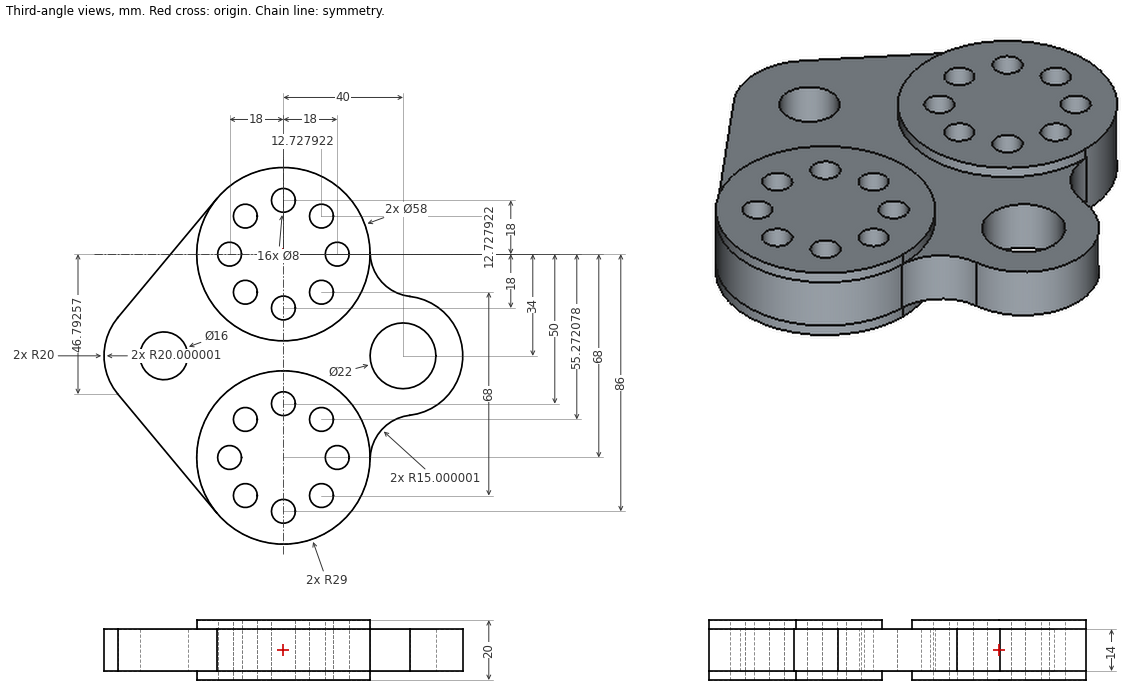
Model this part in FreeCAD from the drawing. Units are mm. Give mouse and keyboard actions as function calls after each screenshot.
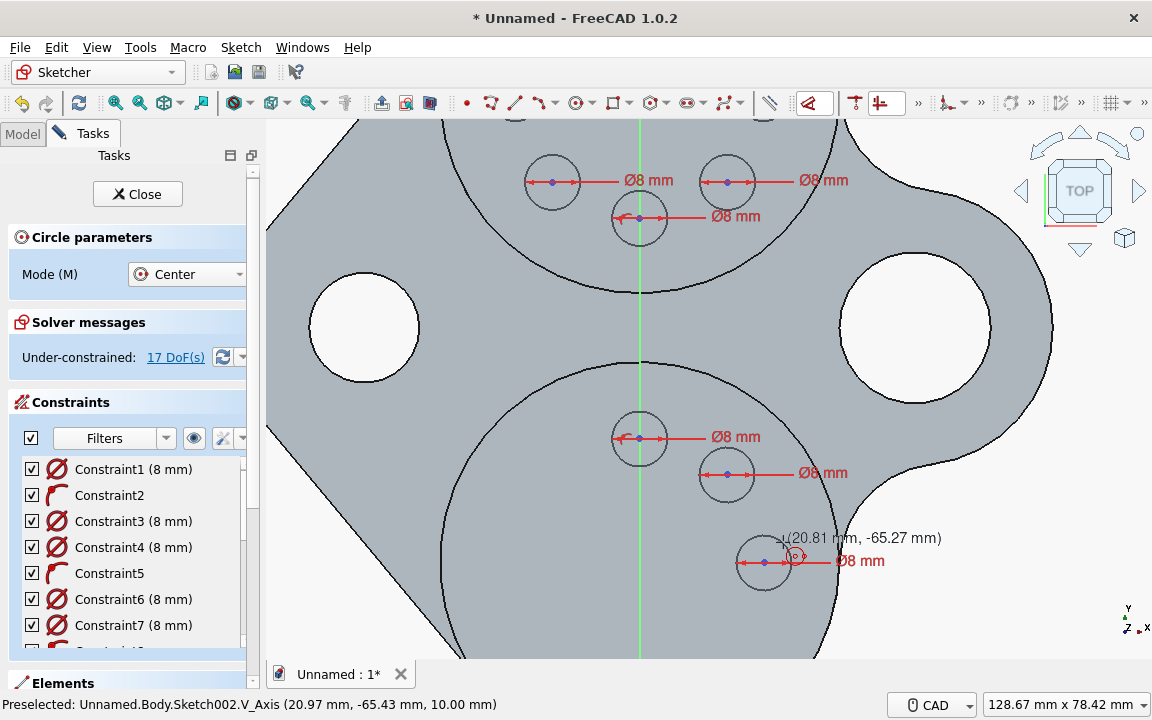
scroll(641, 439, down, 4)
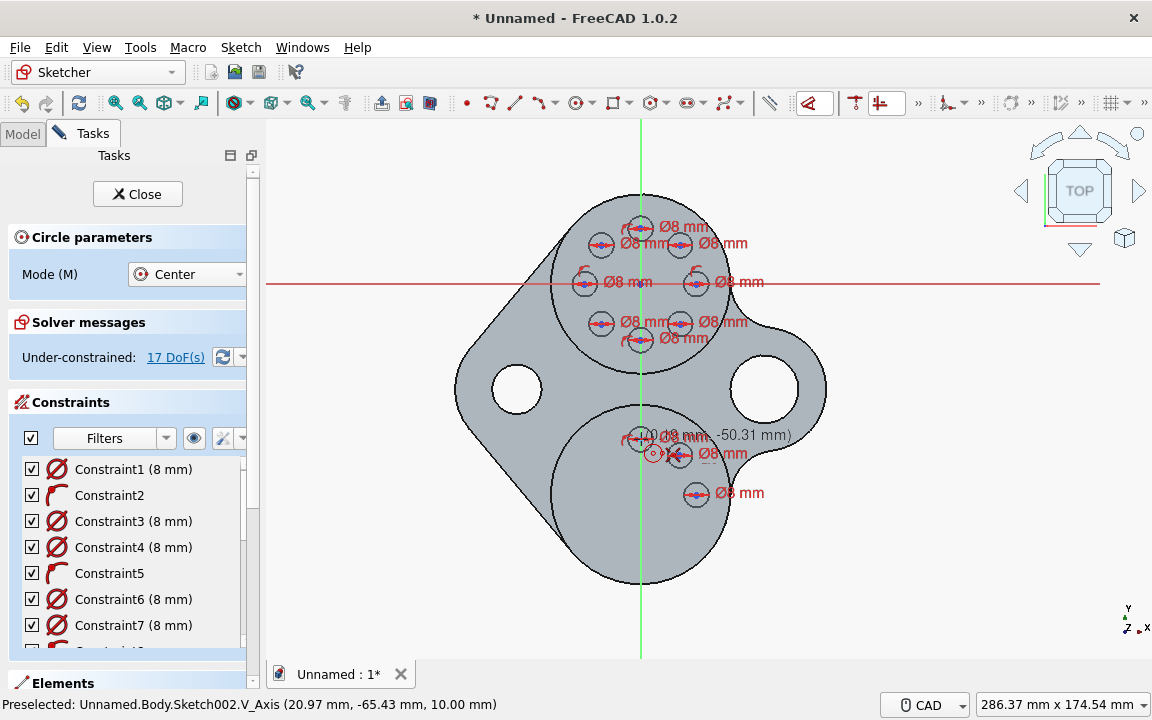
scroll(680, 534, up, 4)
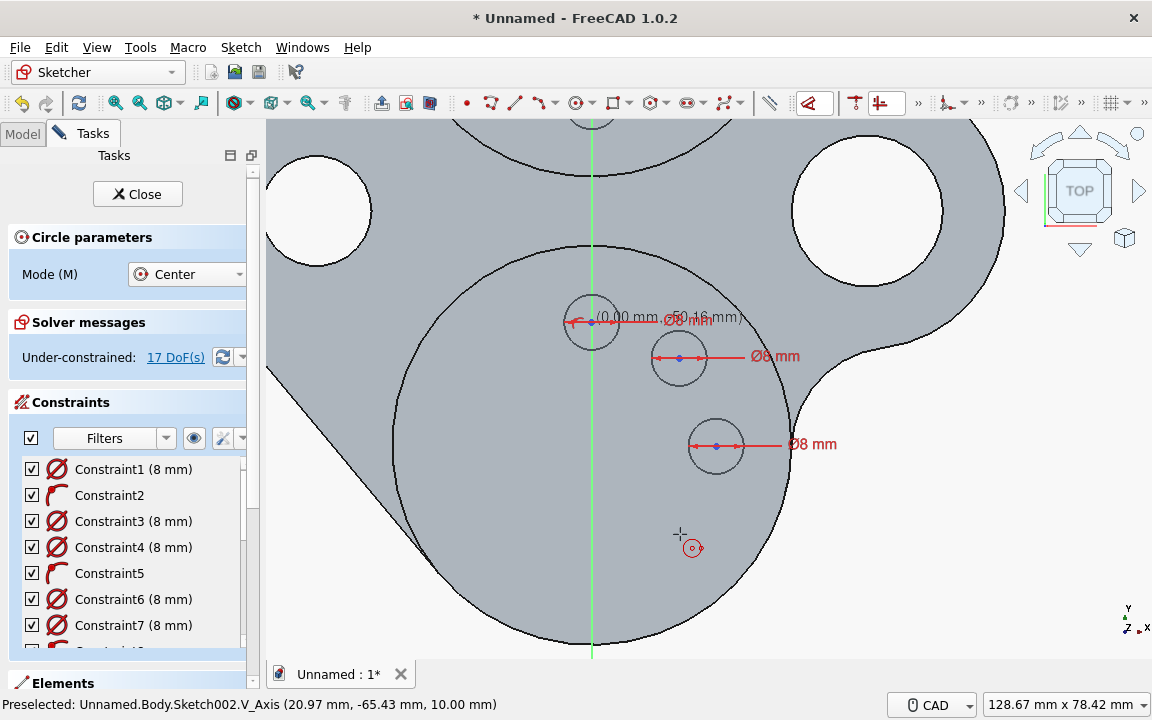
click(679, 533)
move(699, 513)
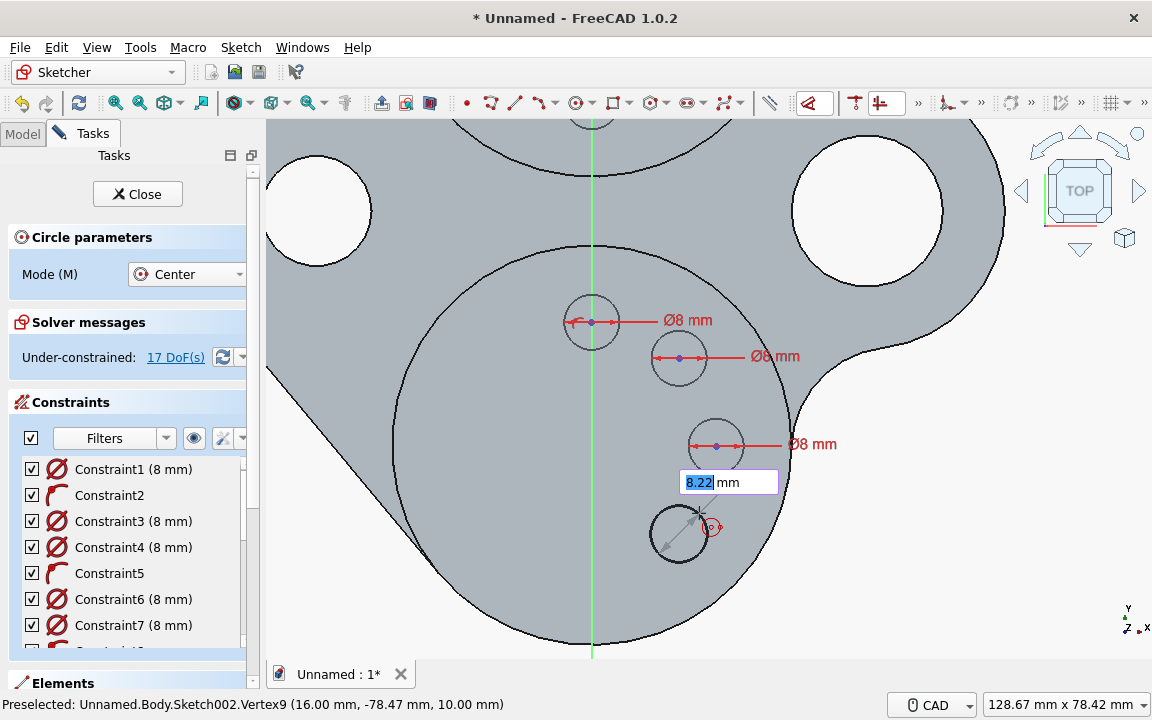
text(8)
key(Return)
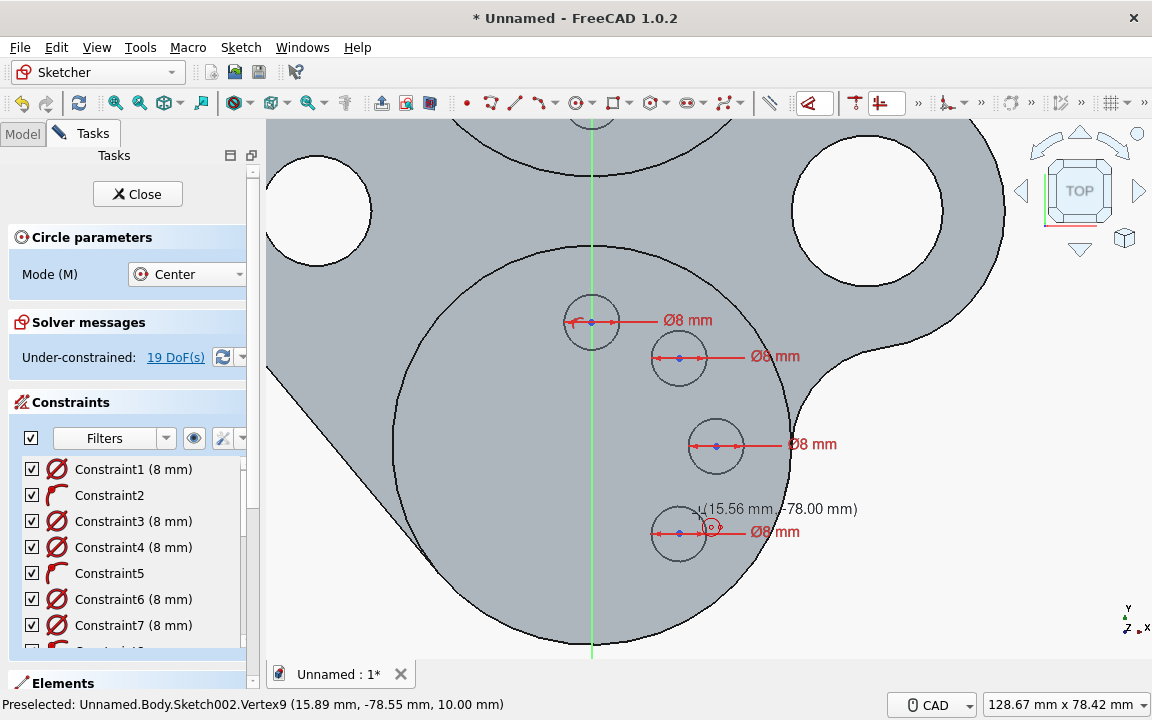
click(592, 569)
move(611, 550)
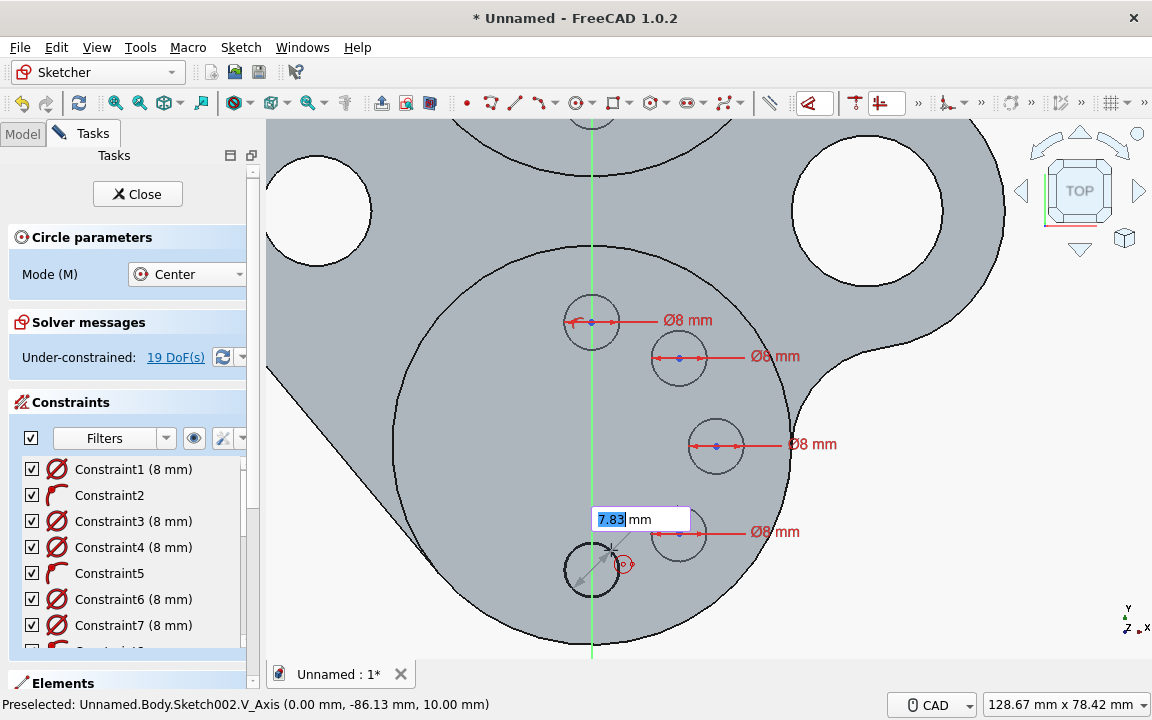
text(8)
key(Return)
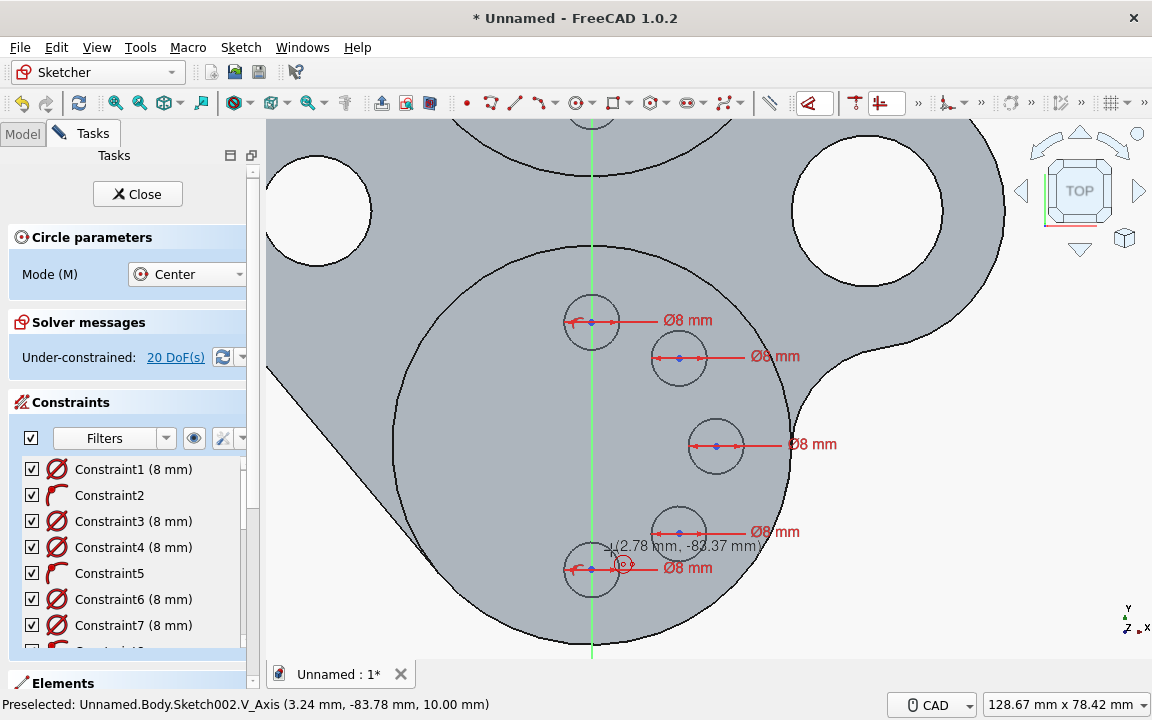
click(504, 533)
move(524, 513)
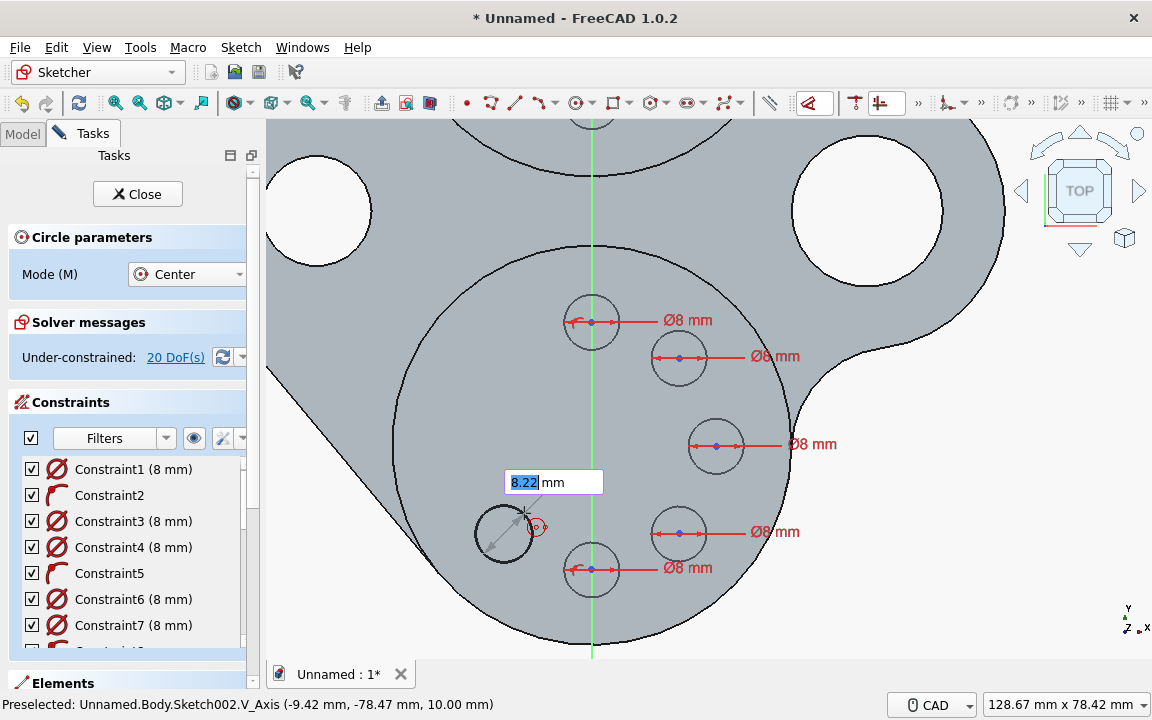
text(8)
key(Return)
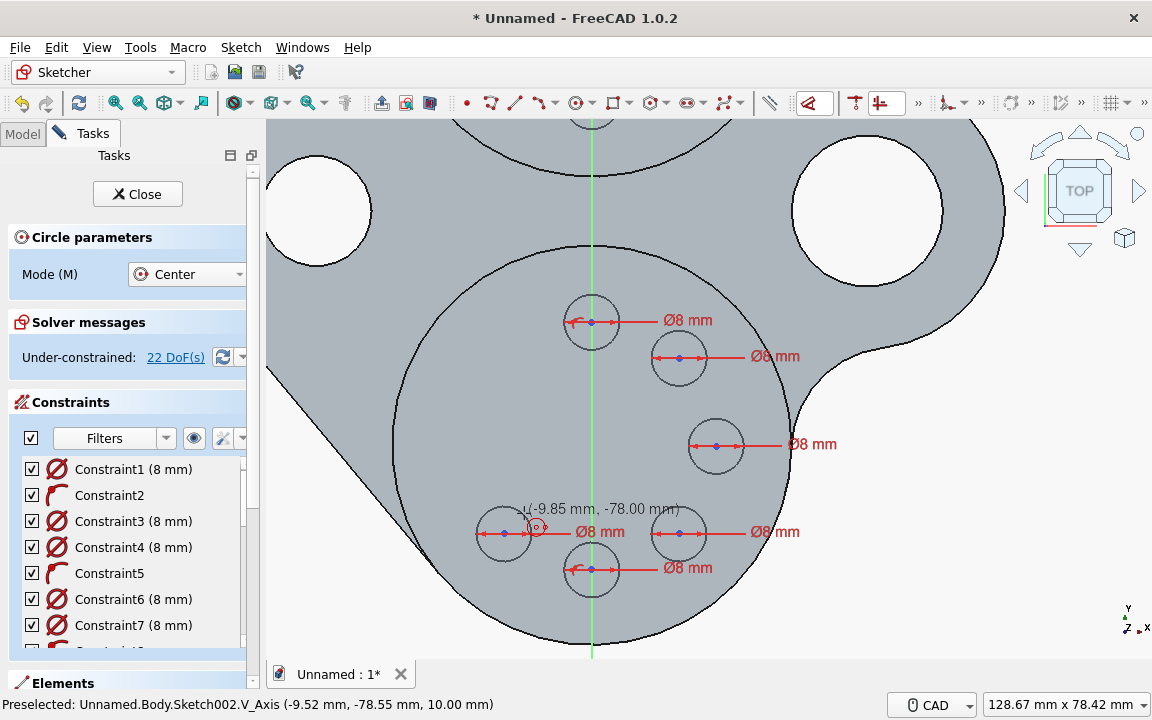
click(468, 445)
move(487, 426)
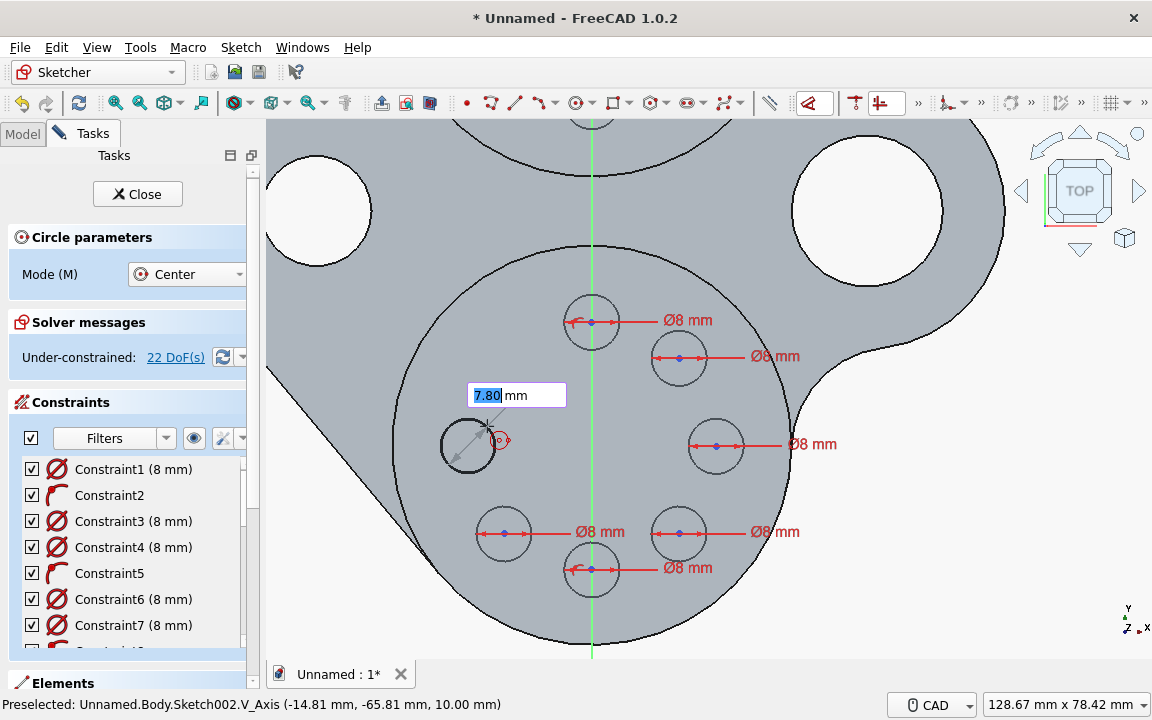
text(8)
key(Return)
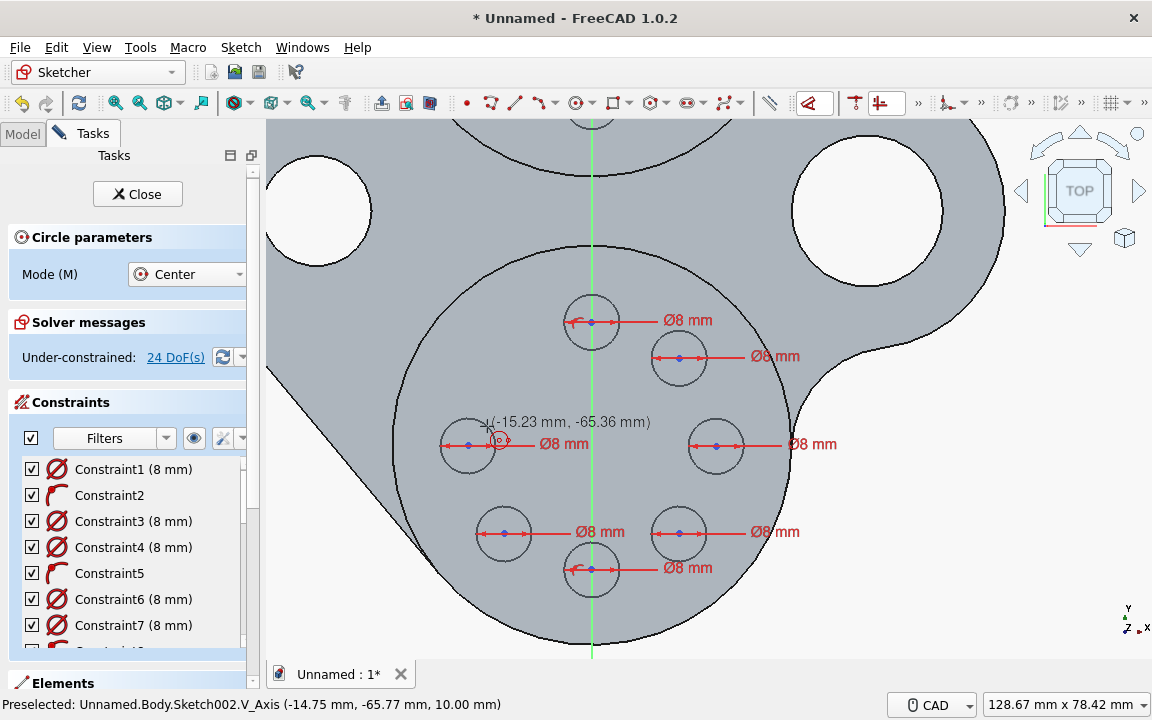
click(504, 358)
move(524, 338)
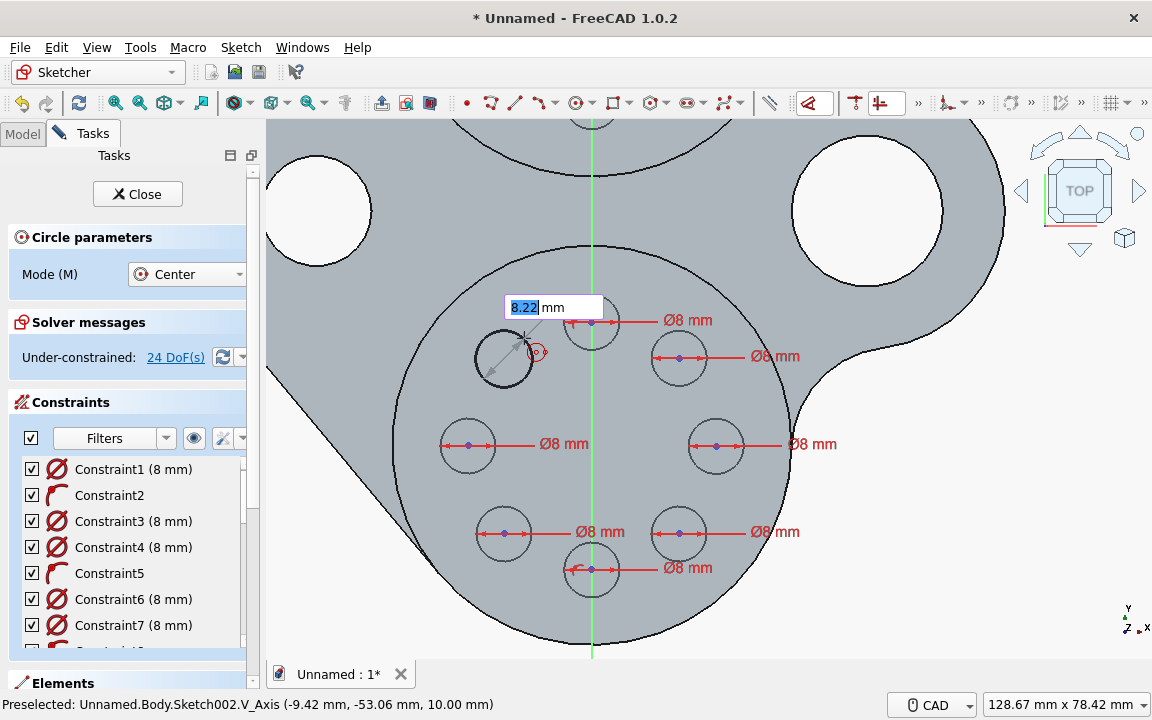
text(8)
key(Return)
key(Escape)